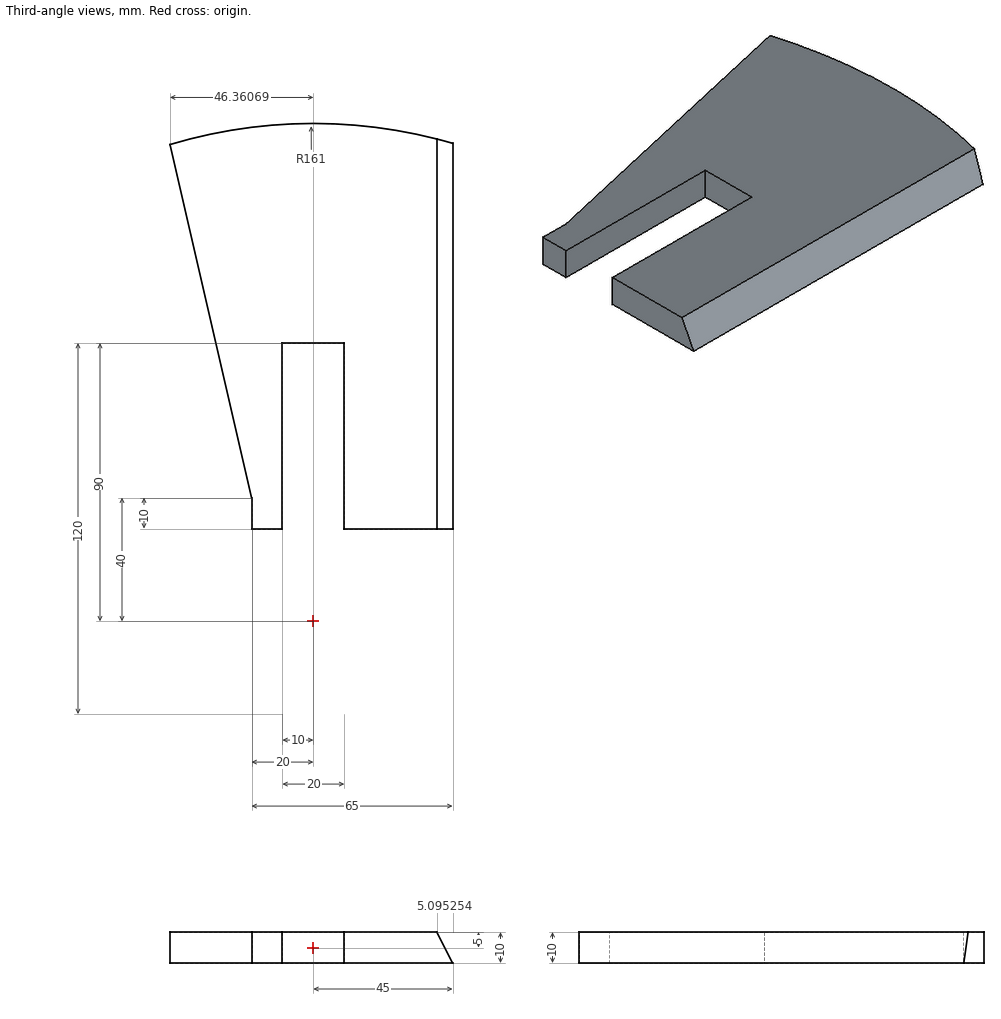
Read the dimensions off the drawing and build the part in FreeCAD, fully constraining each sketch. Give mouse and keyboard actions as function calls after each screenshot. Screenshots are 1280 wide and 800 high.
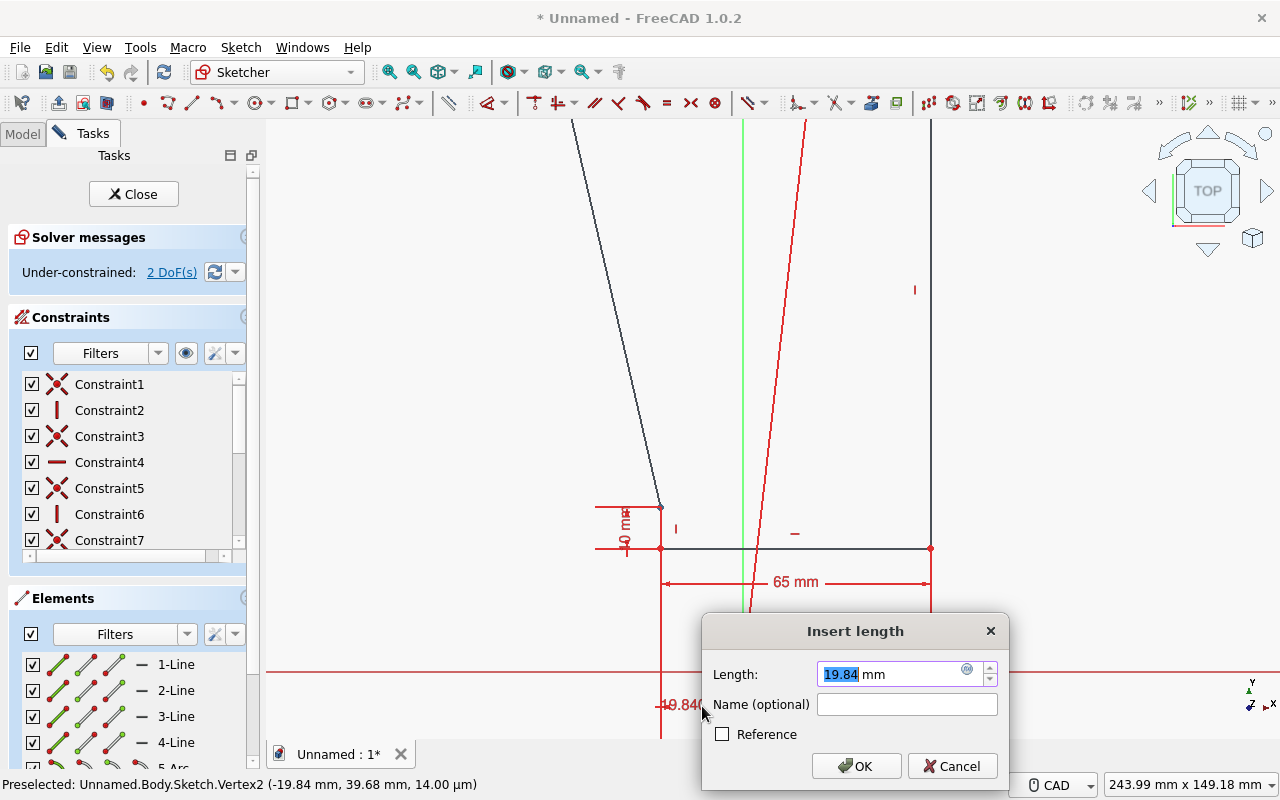
text(20)
key(Return)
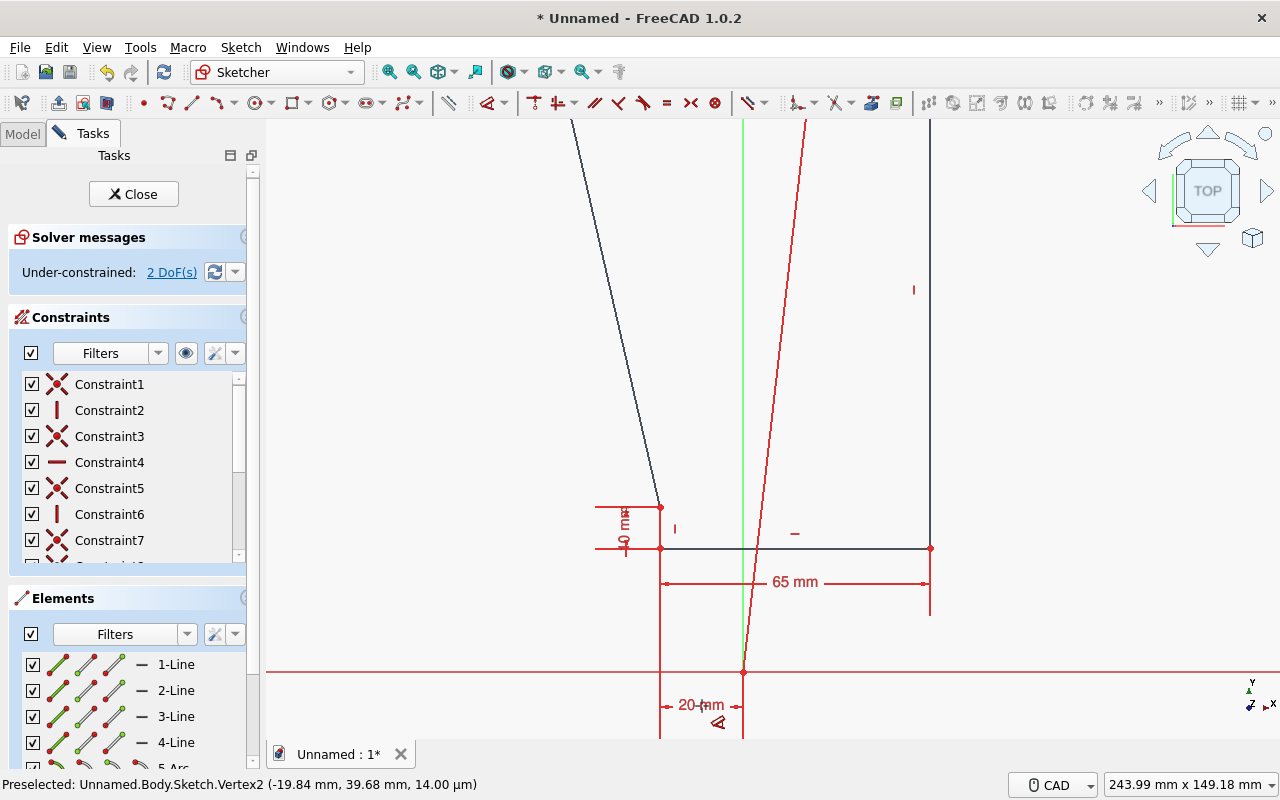
click(660, 507)
click(626, 590)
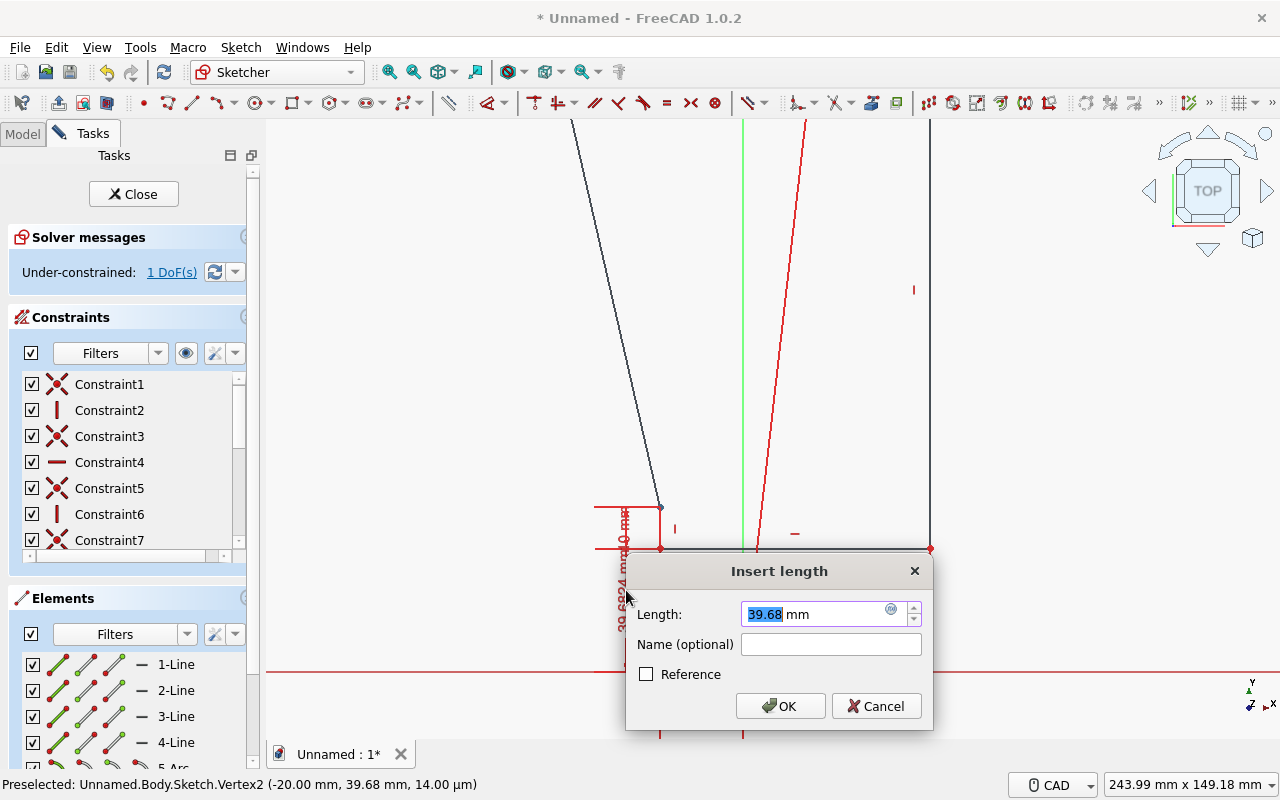
text(40)
key(Return)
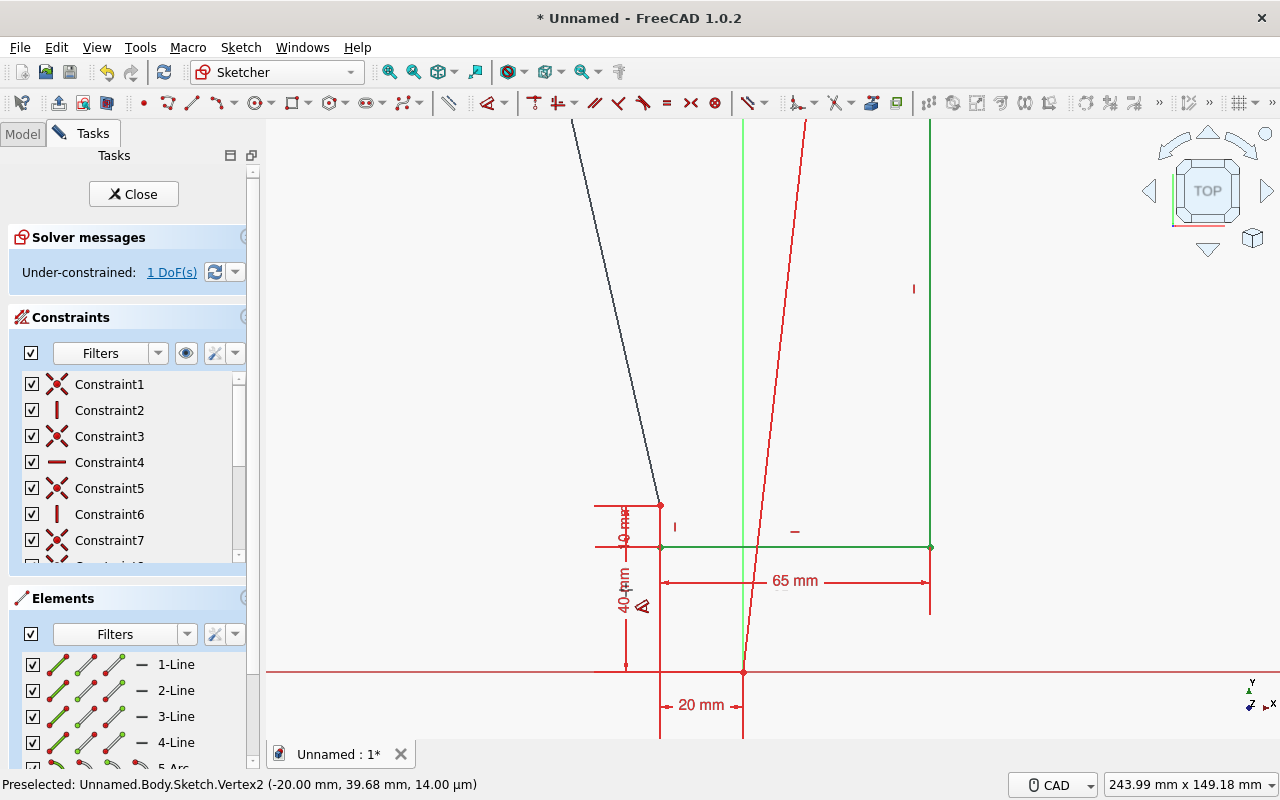
scroll(661, 540, down, 3)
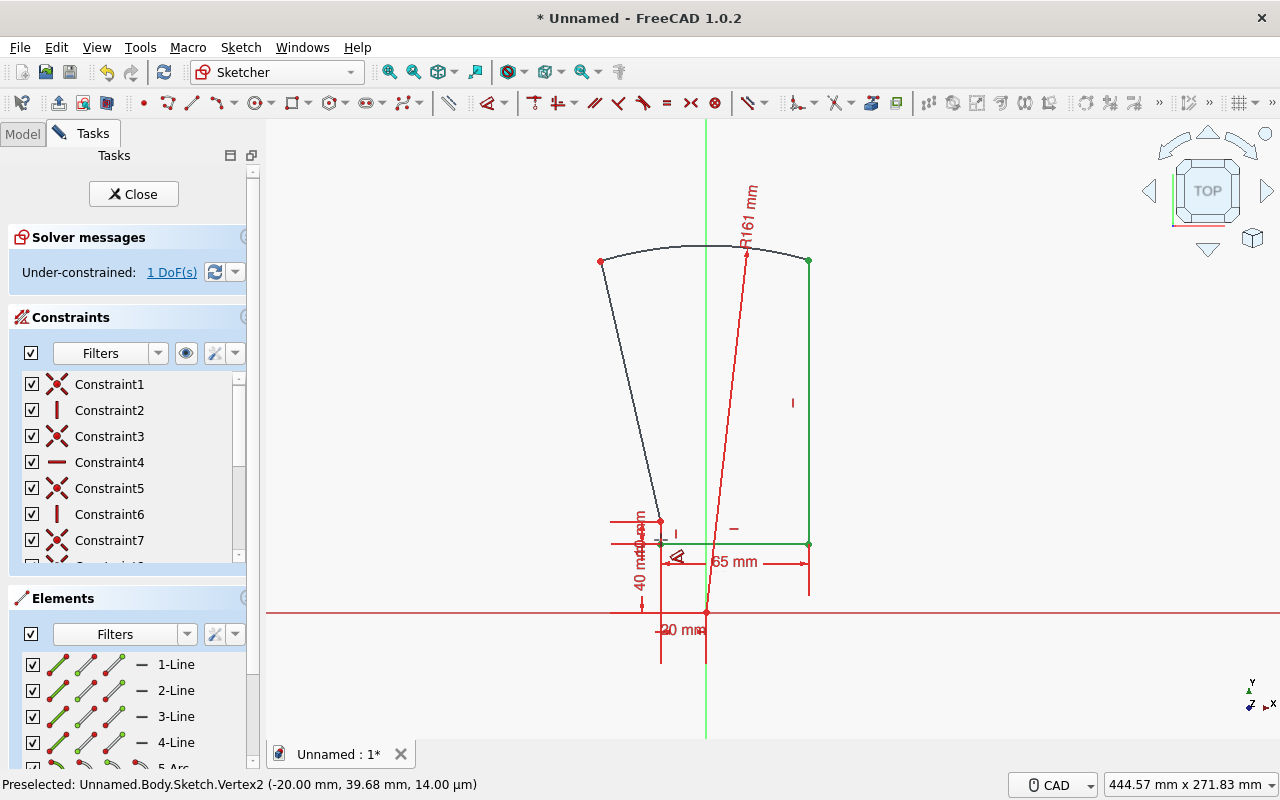
click(601, 261)
click(654, 227)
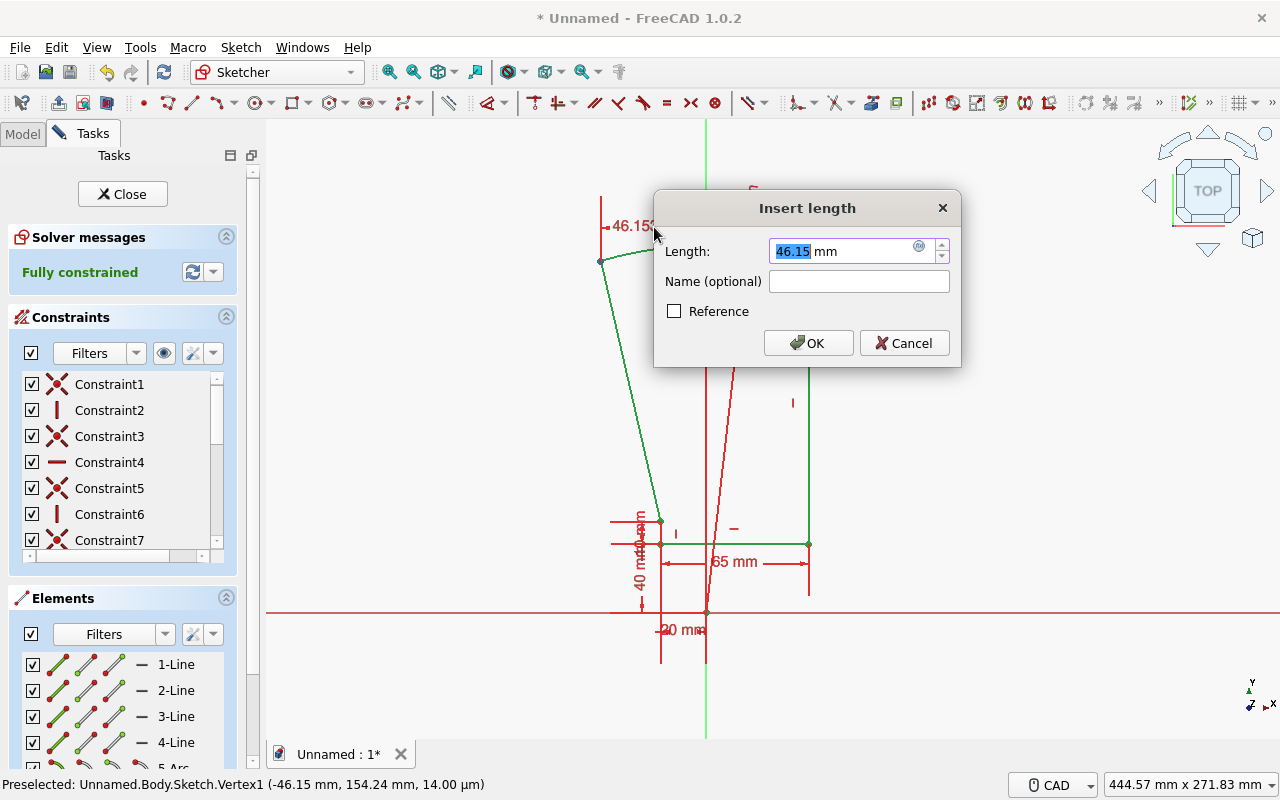
text(46.36069)
key(Return)
key(Escape)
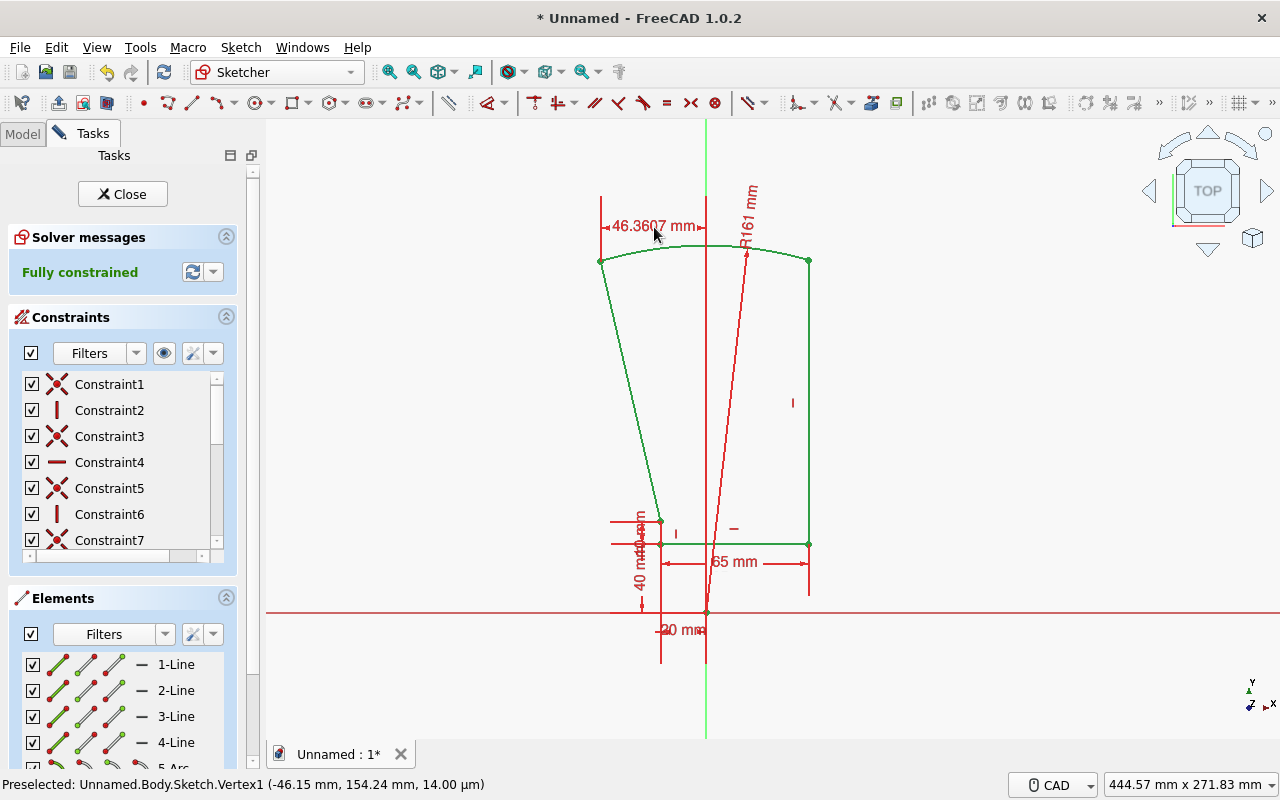
click(123, 194)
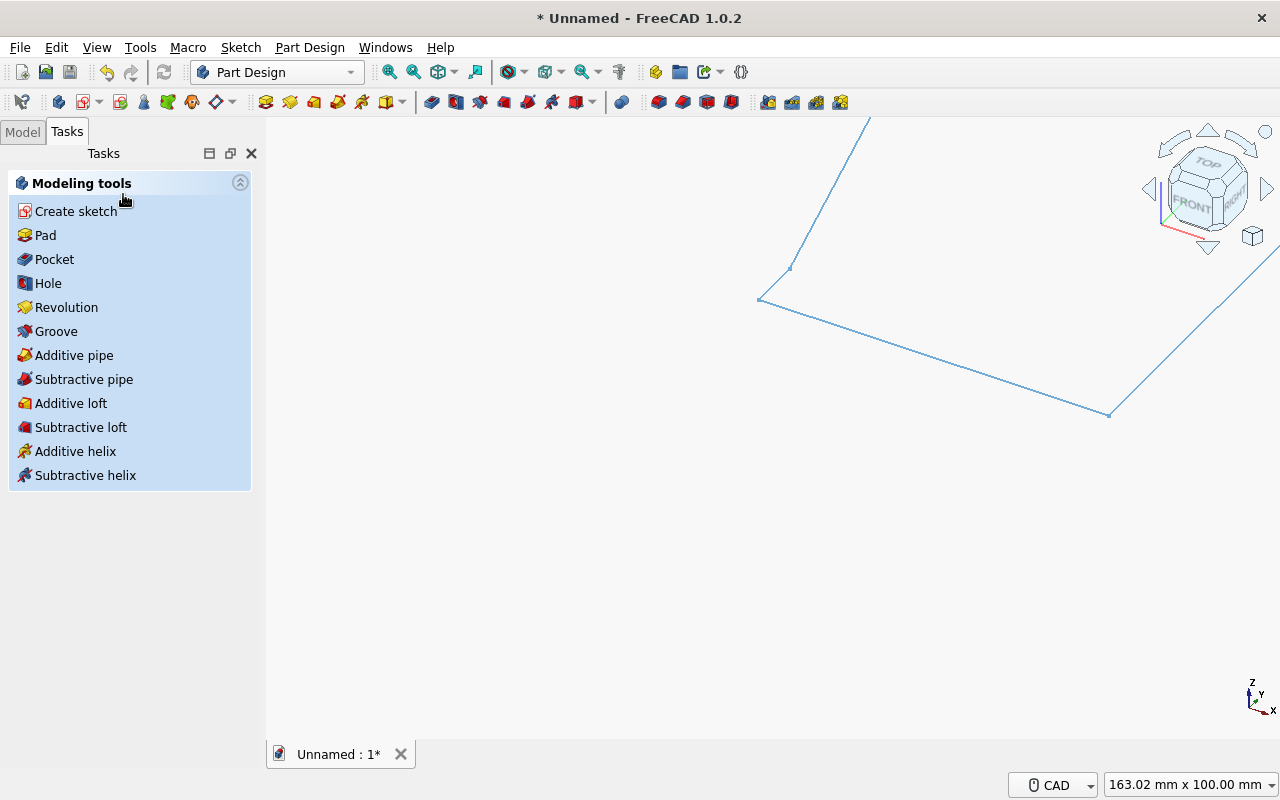
click(266, 102)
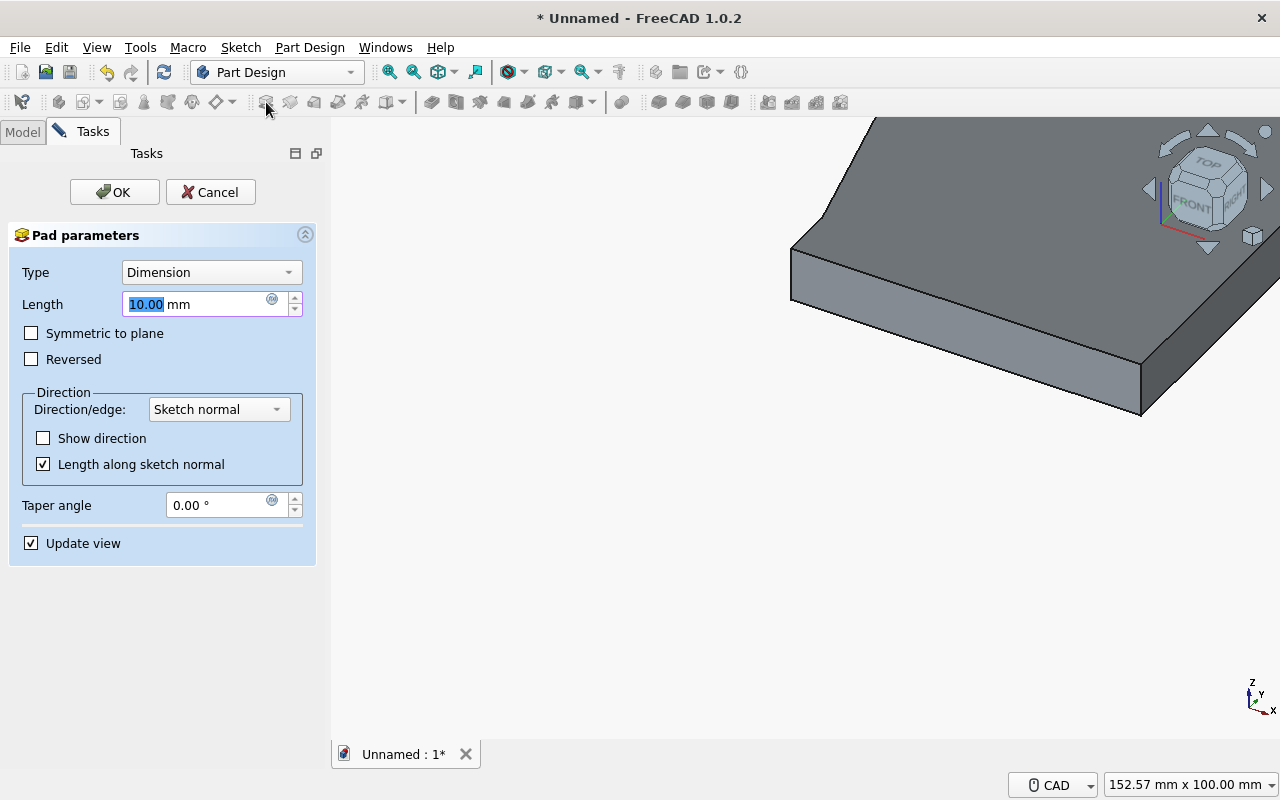
text(10)
key(Tab)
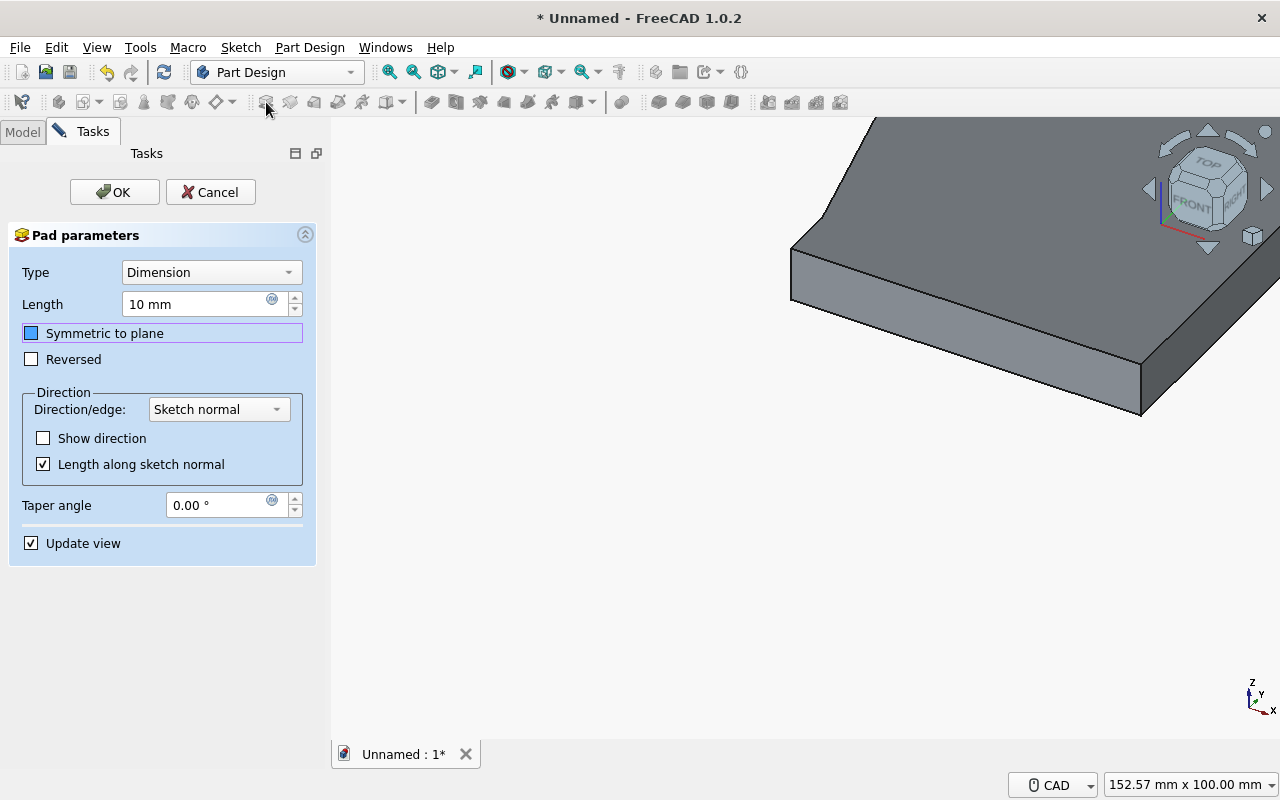
click(30, 333)